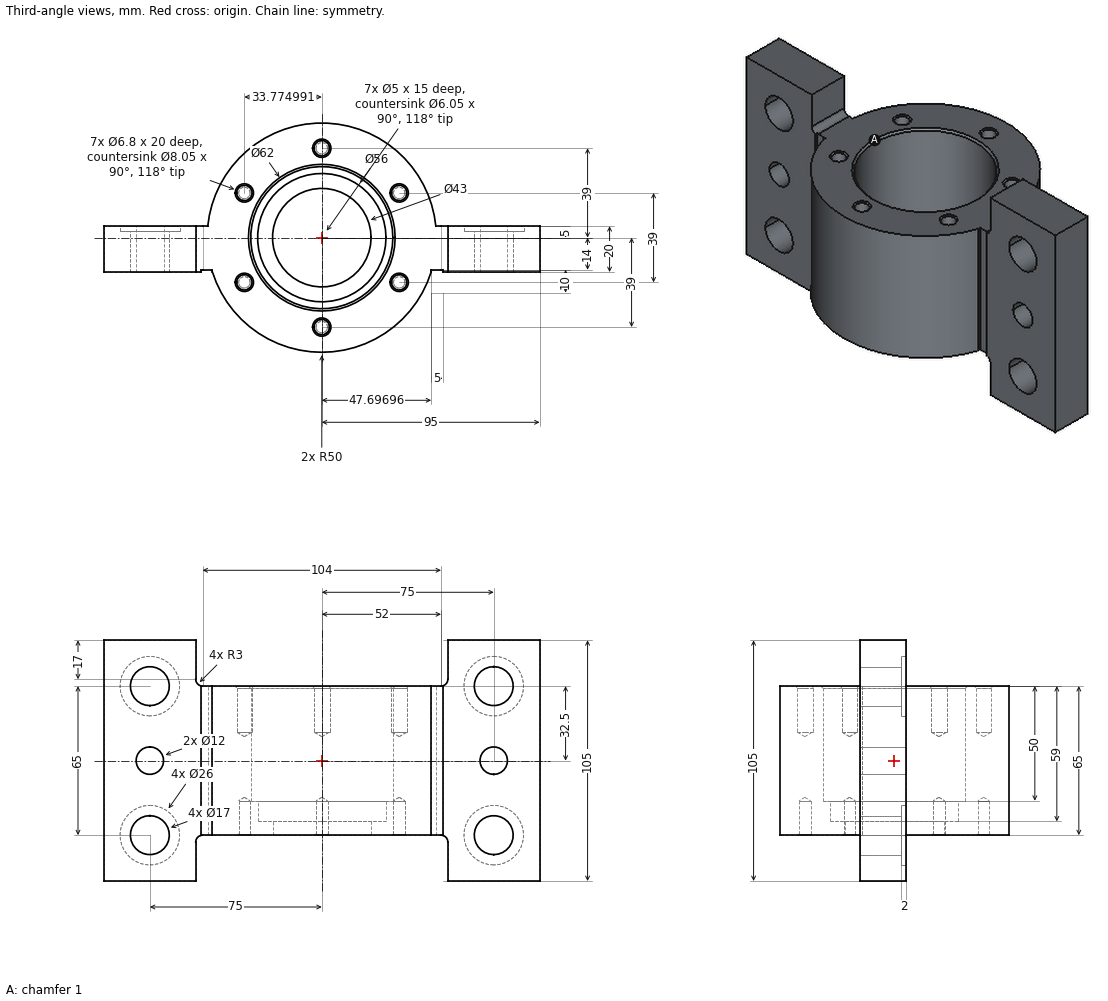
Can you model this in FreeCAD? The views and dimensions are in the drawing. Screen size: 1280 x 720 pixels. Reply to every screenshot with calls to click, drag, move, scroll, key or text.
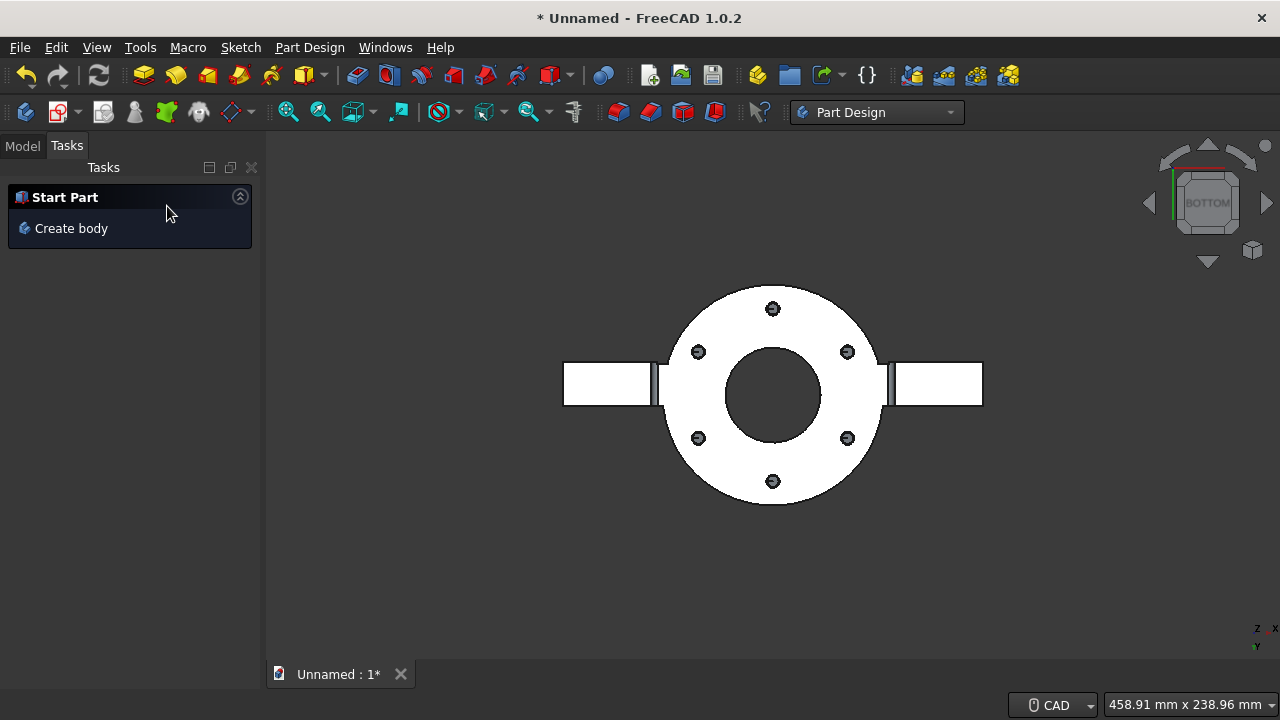
key(0)